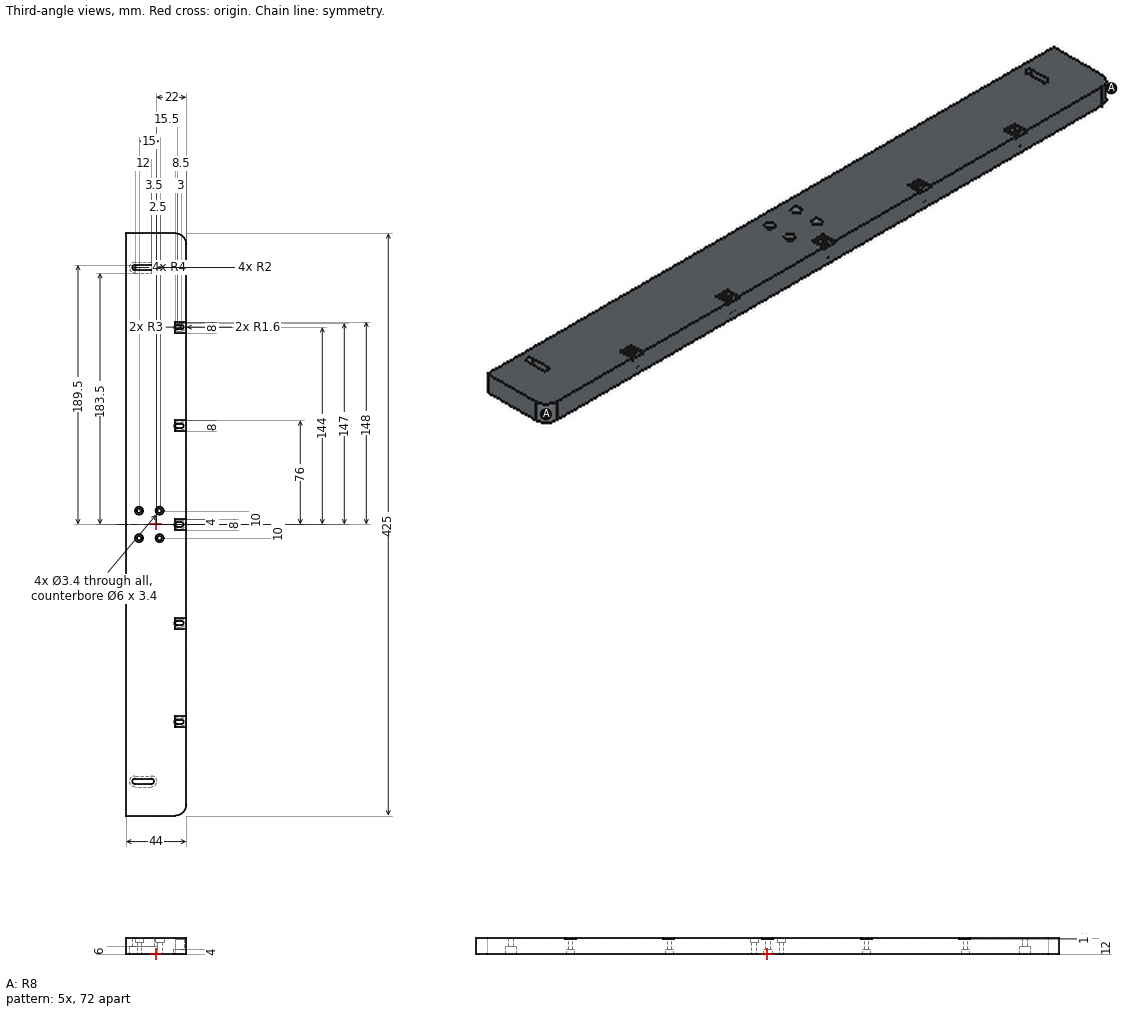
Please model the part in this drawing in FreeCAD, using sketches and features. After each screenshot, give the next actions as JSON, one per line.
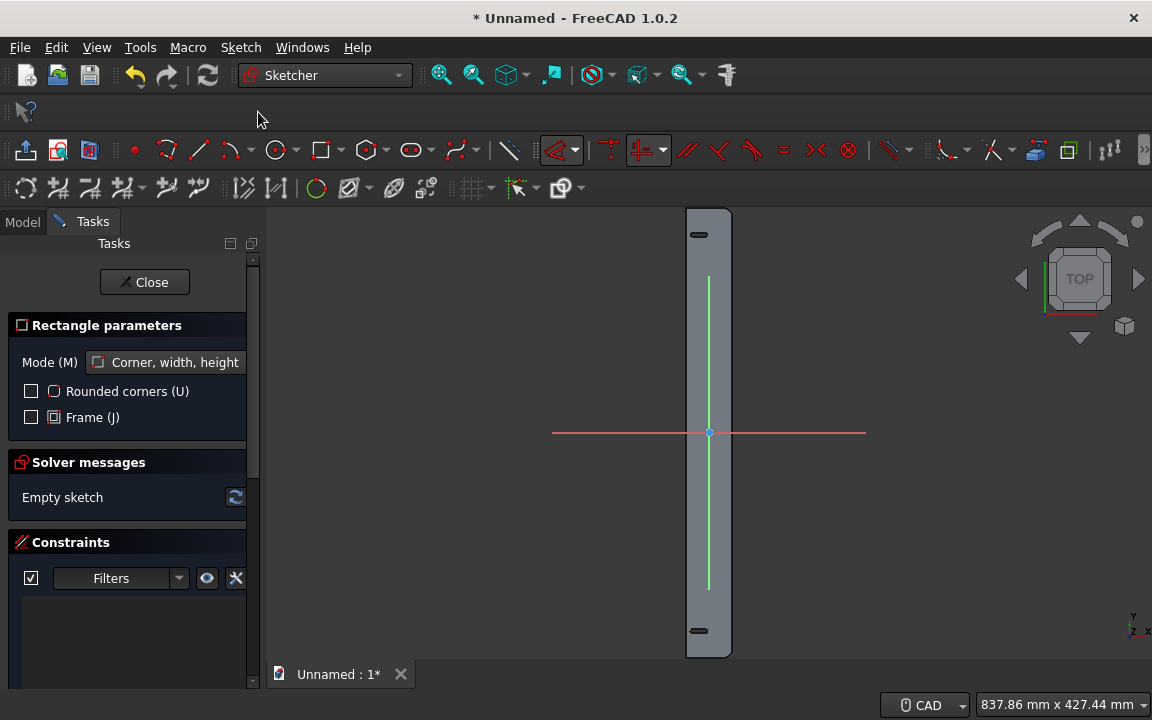
{"action": "scroll", "coordinate": [723, 276], "scroll_direction": "up", "scroll_amount": 4}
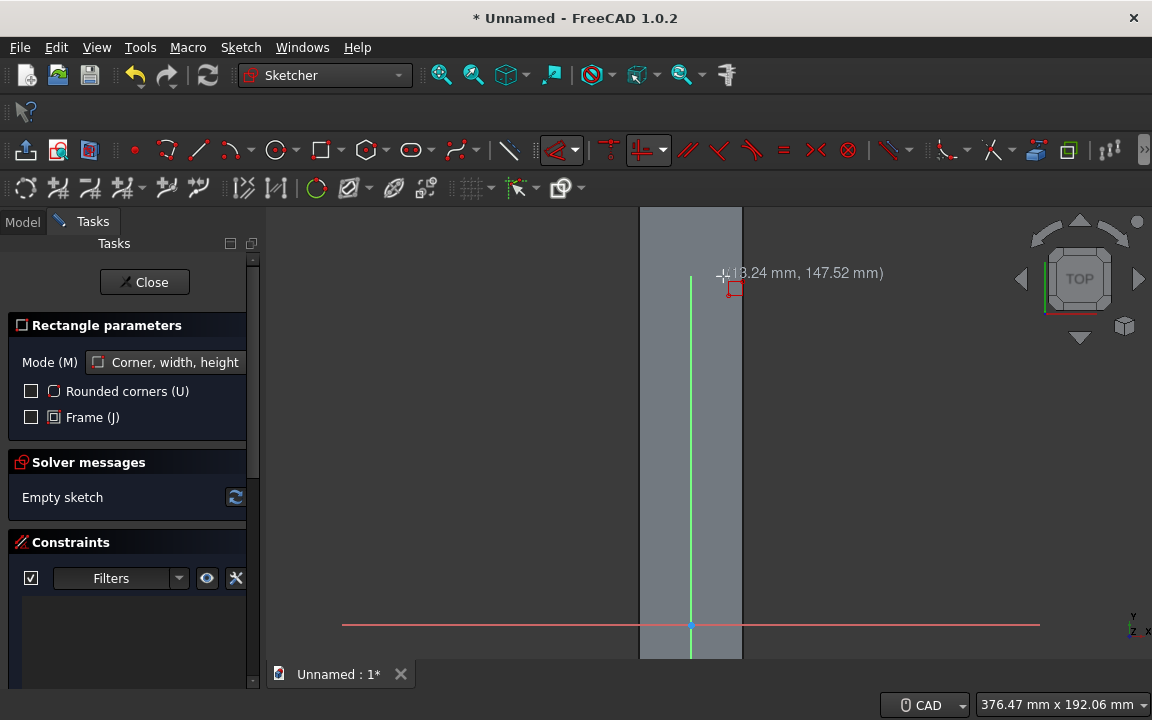
{"action": "left_click", "coordinate": [723, 277]}
{"action": "left_click", "coordinate": [743, 296]}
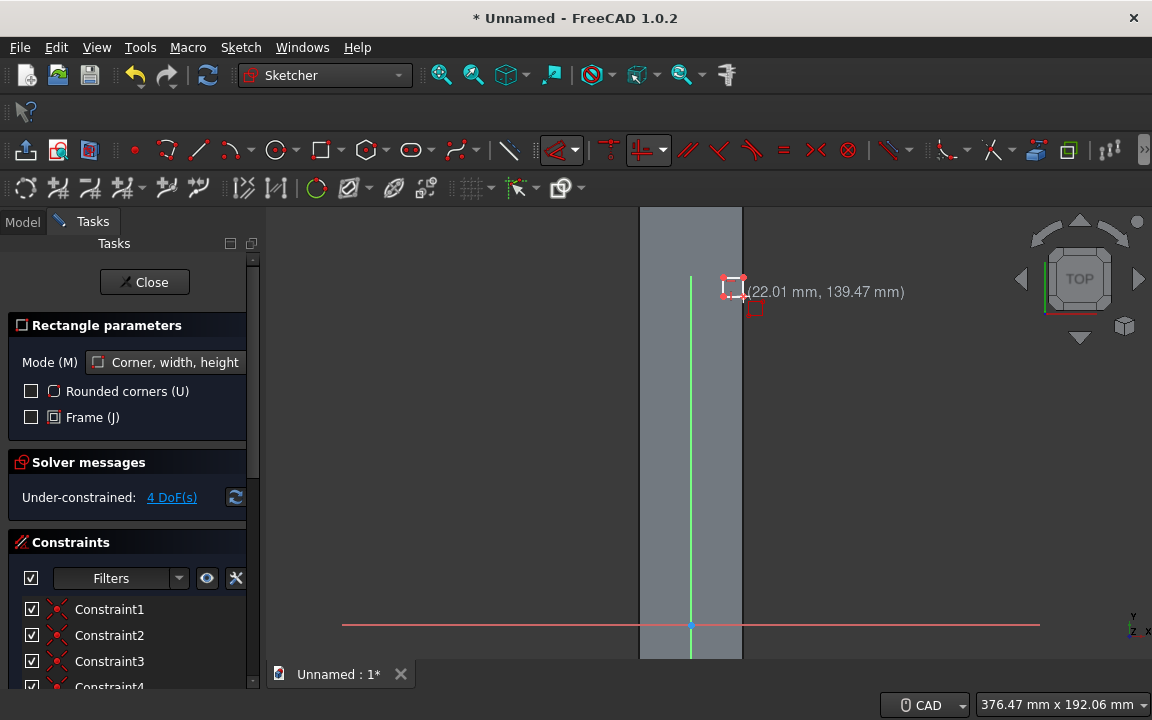
{"action": "left_click", "coordinate": [723, 446]}
{"action": "left_click", "coordinate": [743, 465]}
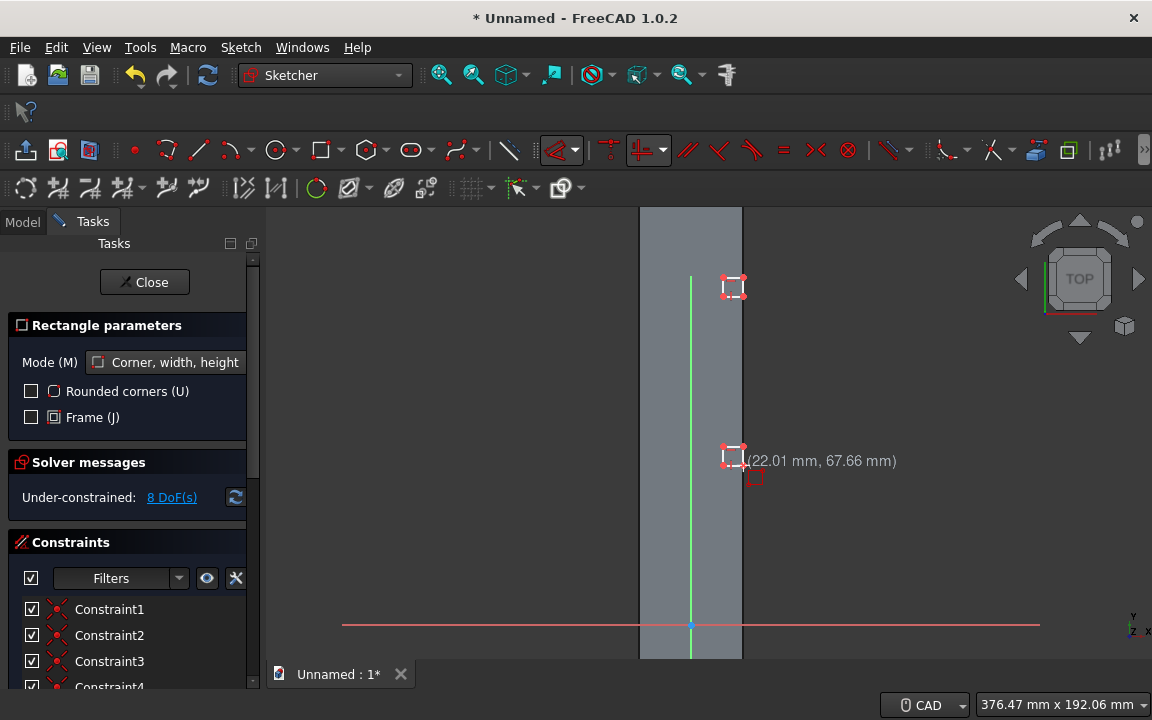
{"action": "scroll", "coordinate": [723, 616], "scroll_direction": "up", "scroll_amount": 3}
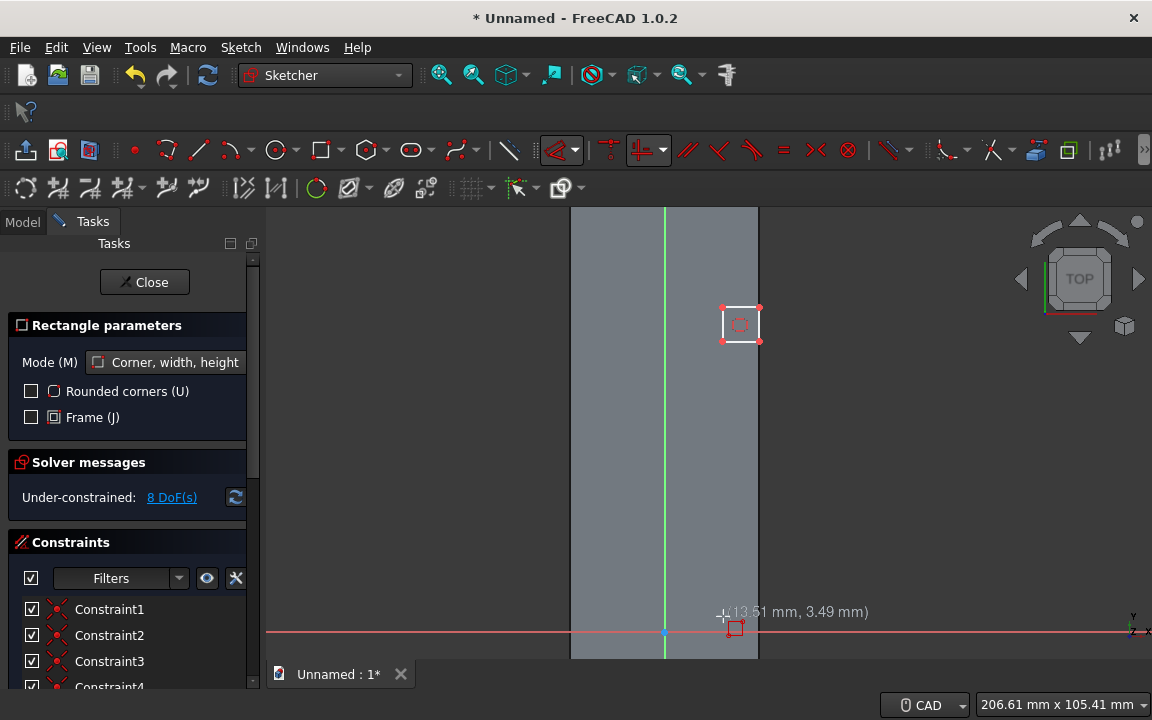
{"action": "left_click", "coordinate": [723, 615]}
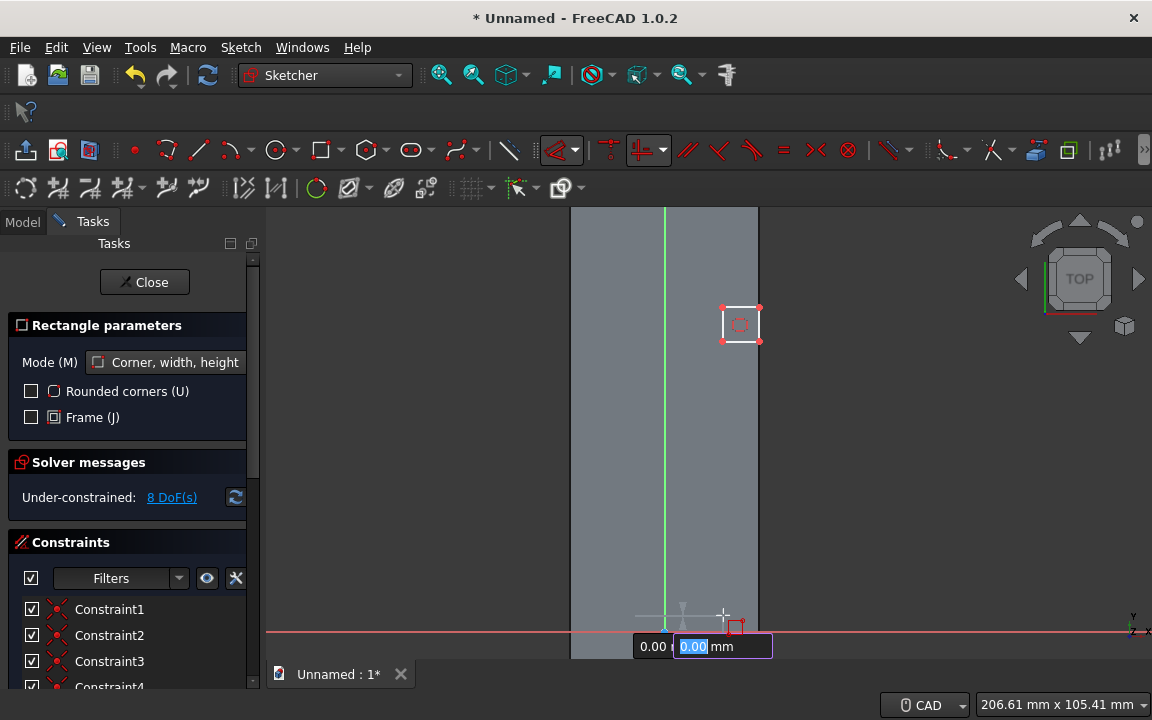
{"action": "scroll", "coordinate": [622, 383], "scroll_direction": "down", "scroll_amount": 8}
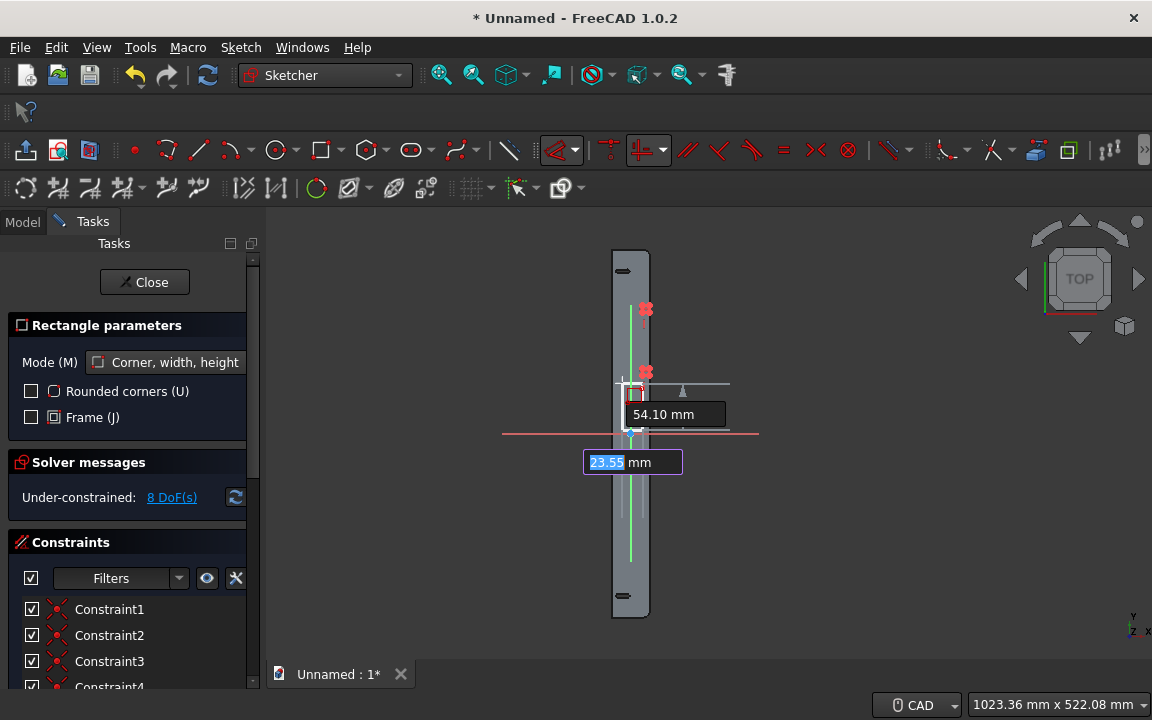
{"action": "scroll", "coordinate": [650, 437], "scroll_direction": "up", "scroll_amount": 8}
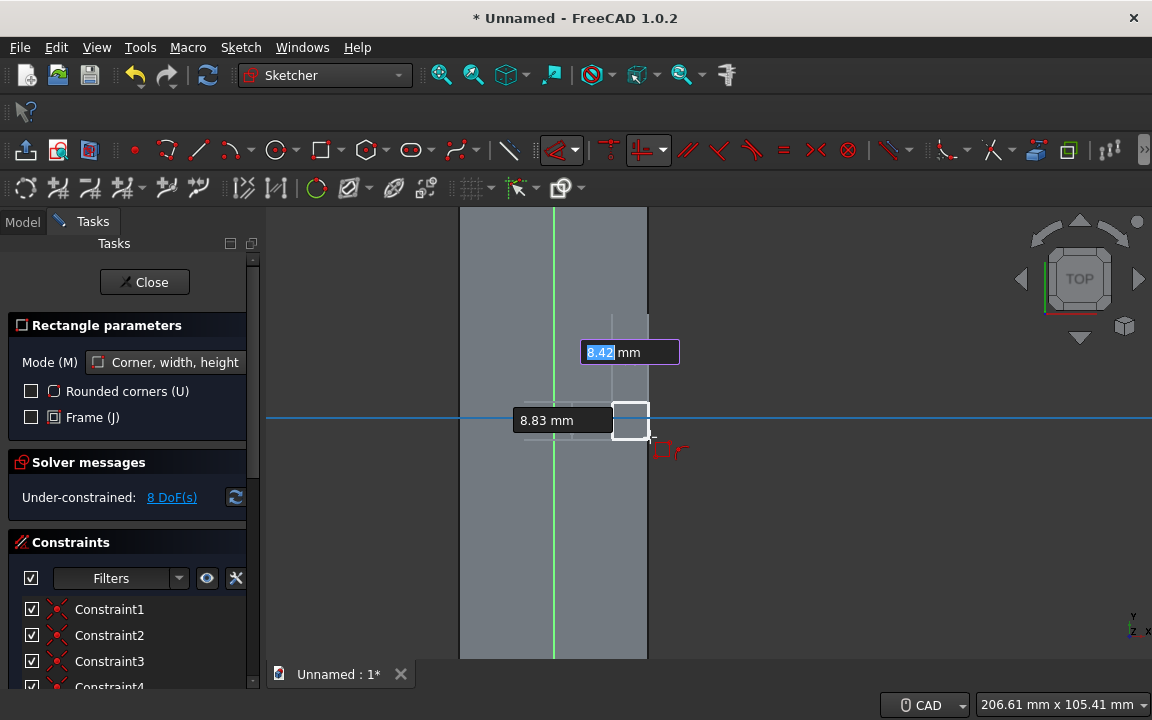
{"action": "left_click", "coordinate": [648, 435]}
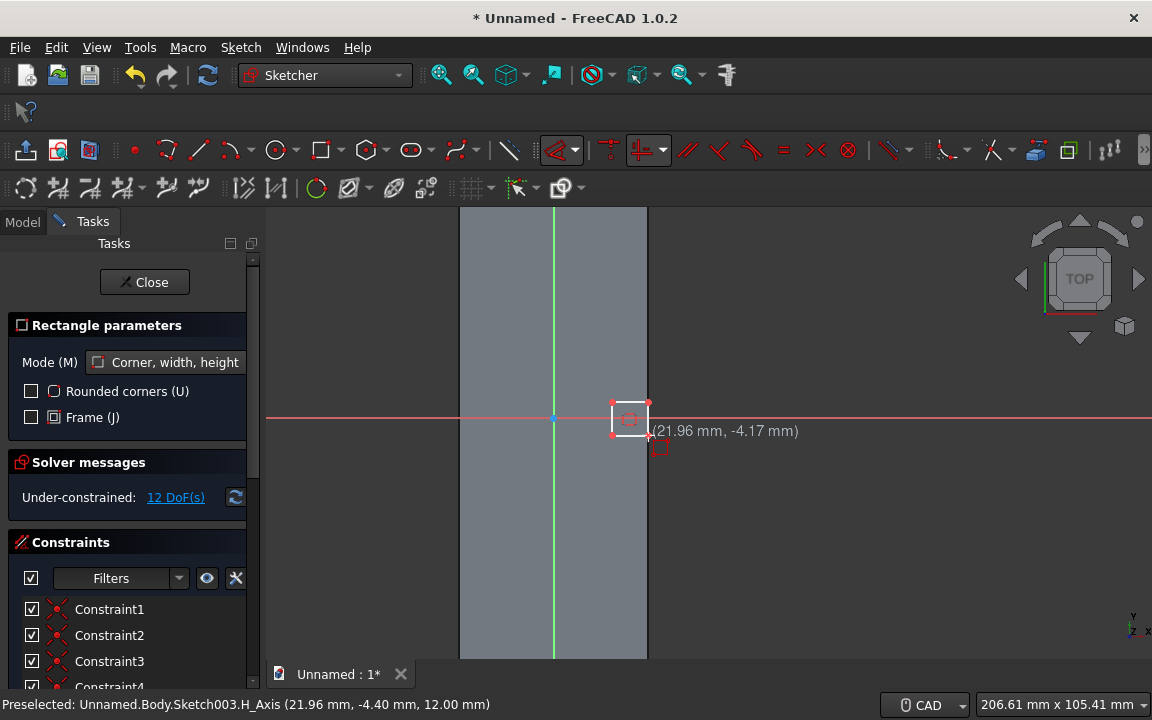
{"action": "scroll", "coordinate": [650, 437], "scroll_direction": "down", "scroll_amount": 8}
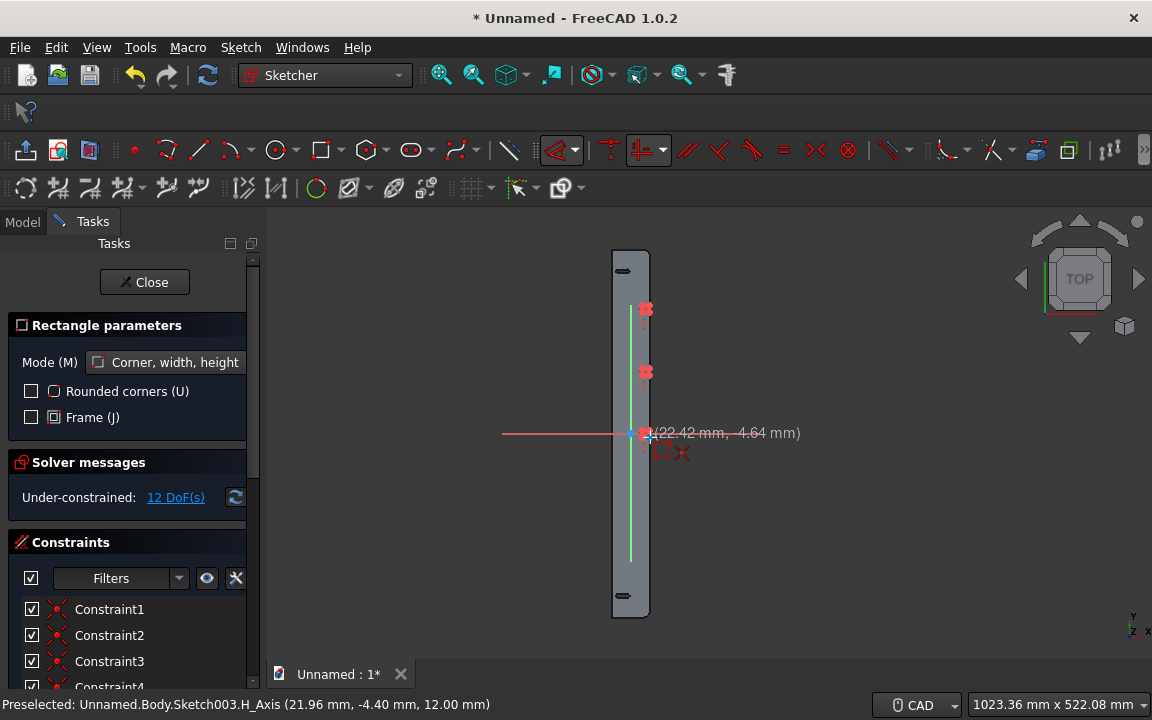
{"action": "scroll", "coordinate": [643, 492], "scroll_direction": "up", "scroll_amount": 5}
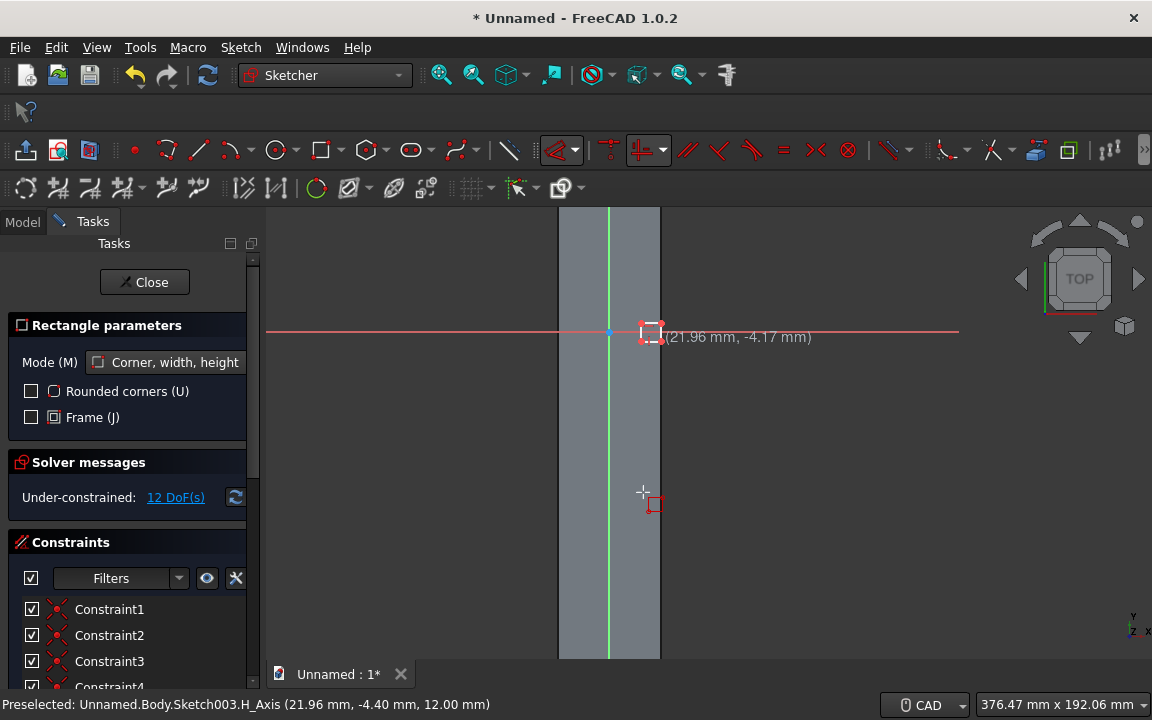
{"action": "left_click", "coordinate": [641, 492]}
{"action": "left_click", "coordinate": [661, 511]}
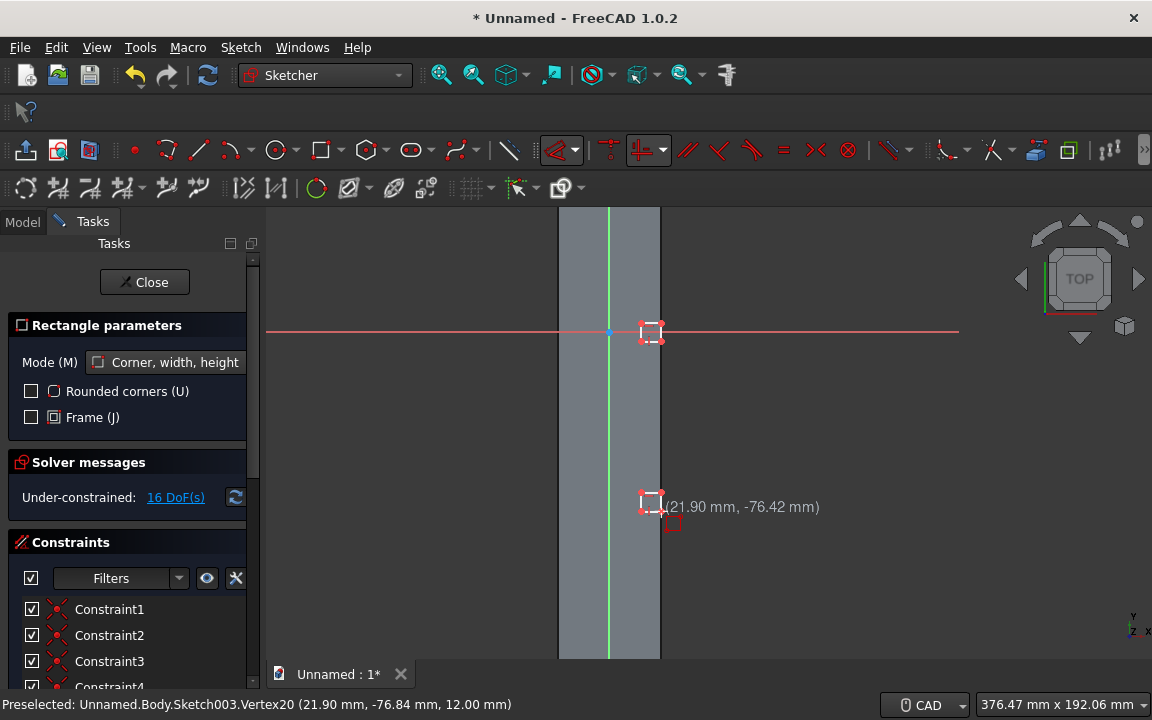
{"action": "scroll", "coordinate": [643, 492], "scroll_direction": "down", "scroll_amount": 5}